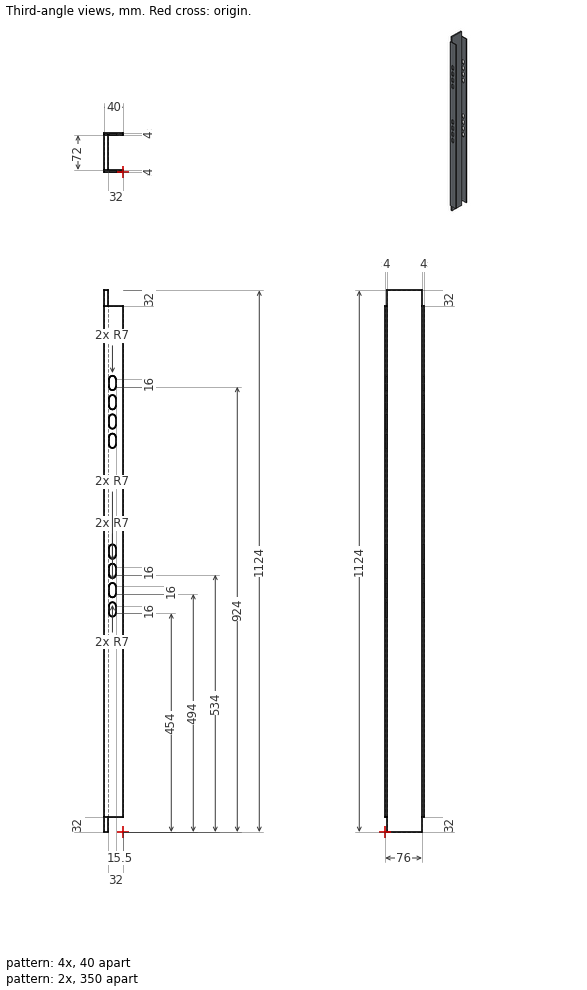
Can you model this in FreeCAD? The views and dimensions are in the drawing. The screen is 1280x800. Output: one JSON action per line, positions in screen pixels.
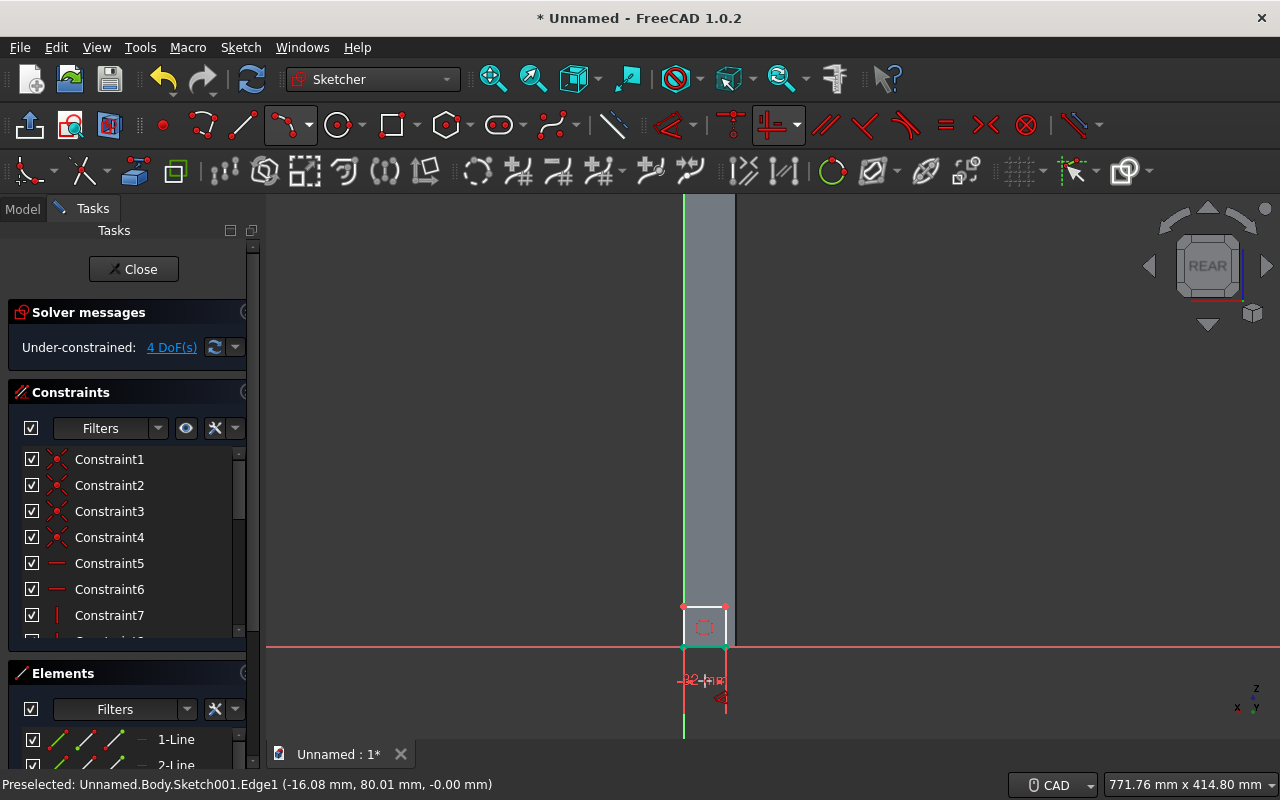
{"action": "left_click", "coordinate": [726, 635]}
{"action": "left_click", "coordinate": [760, 627]}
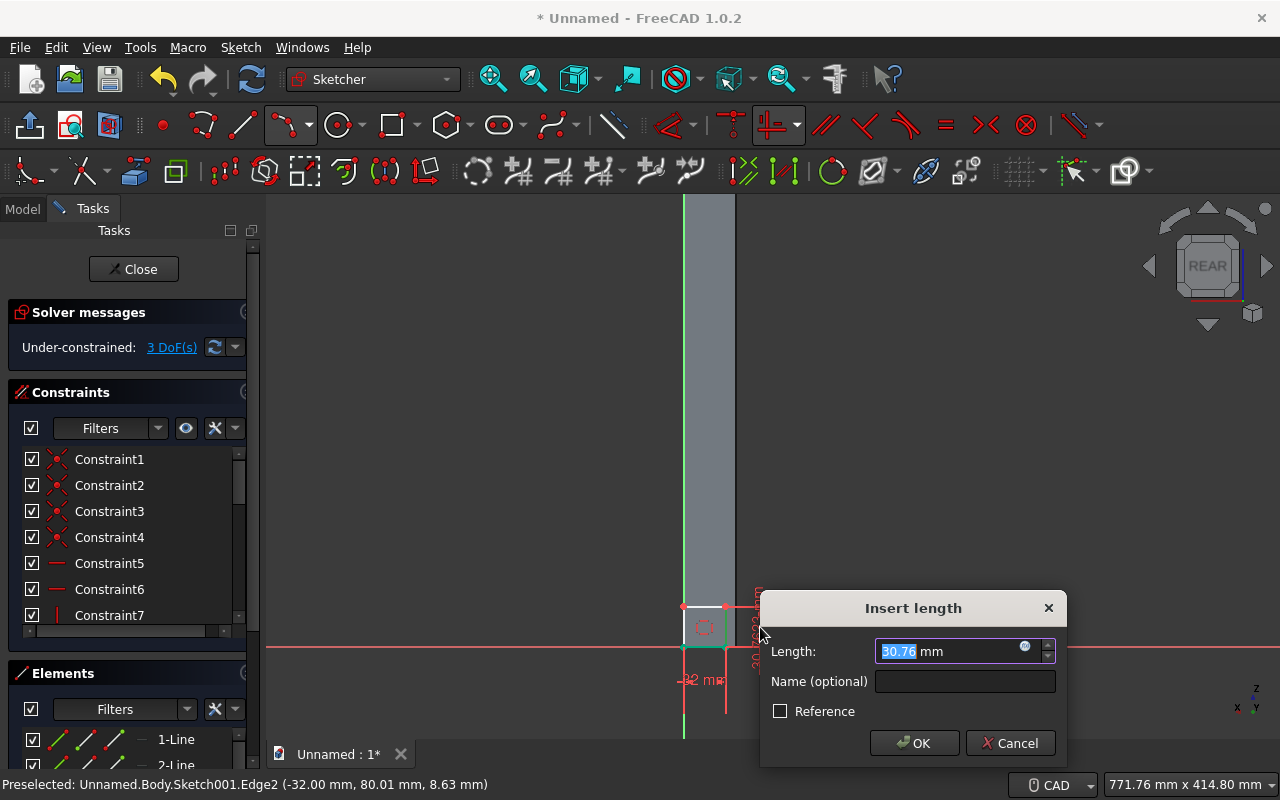
{"action": "type", "text": "32"}
{"action": "key", "text": "Return"}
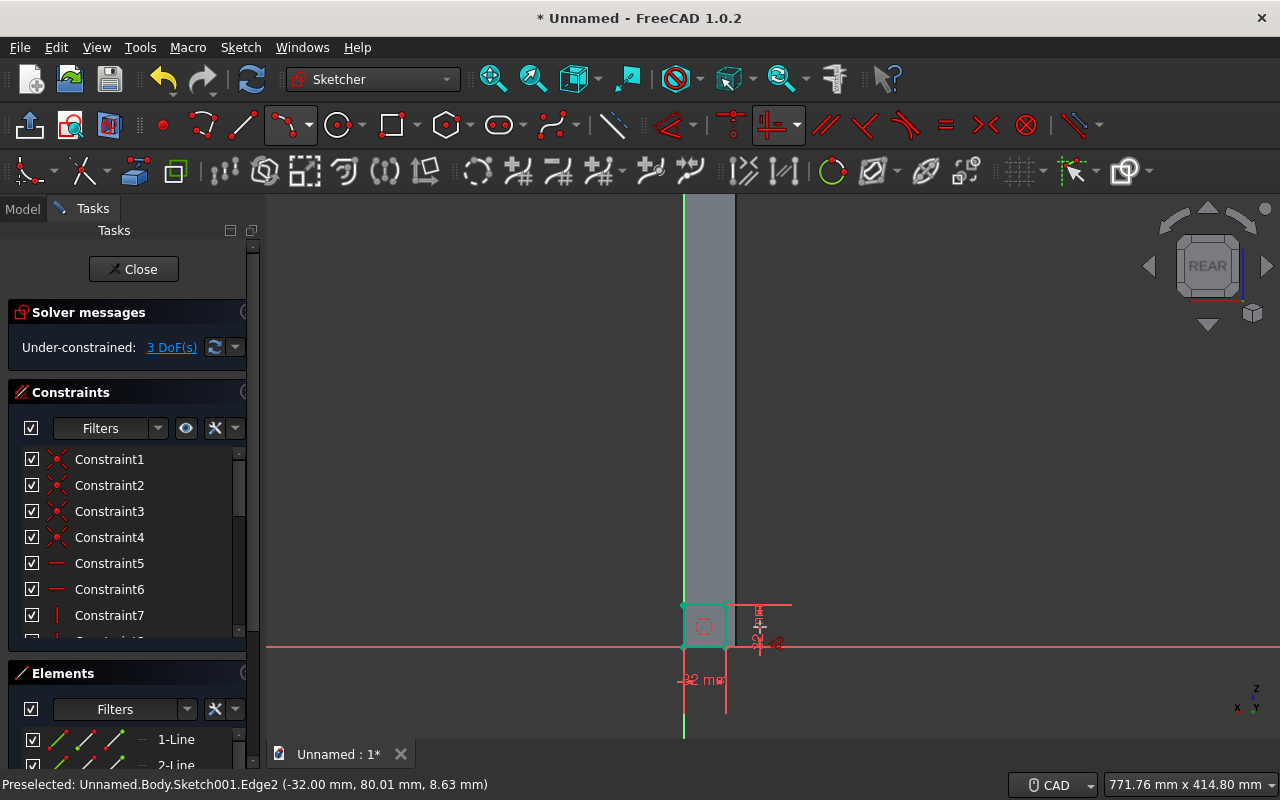
{"action": "scroll", "coordinate": [704, 649], "scroll_direction": "down", "scroll_amount": 7}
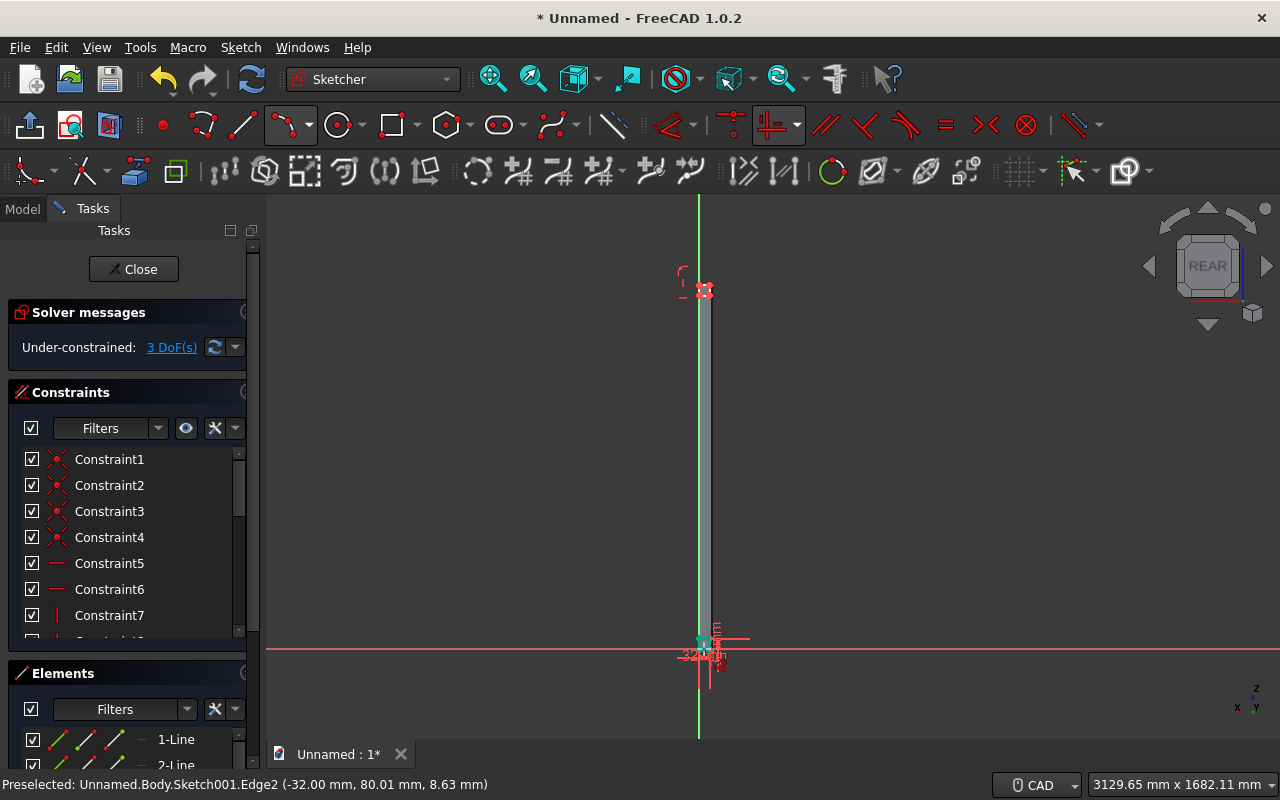
{"action": "scroll", "coordinate": [699, 289], "scroll_direction": "up", "scroll_amount": 8}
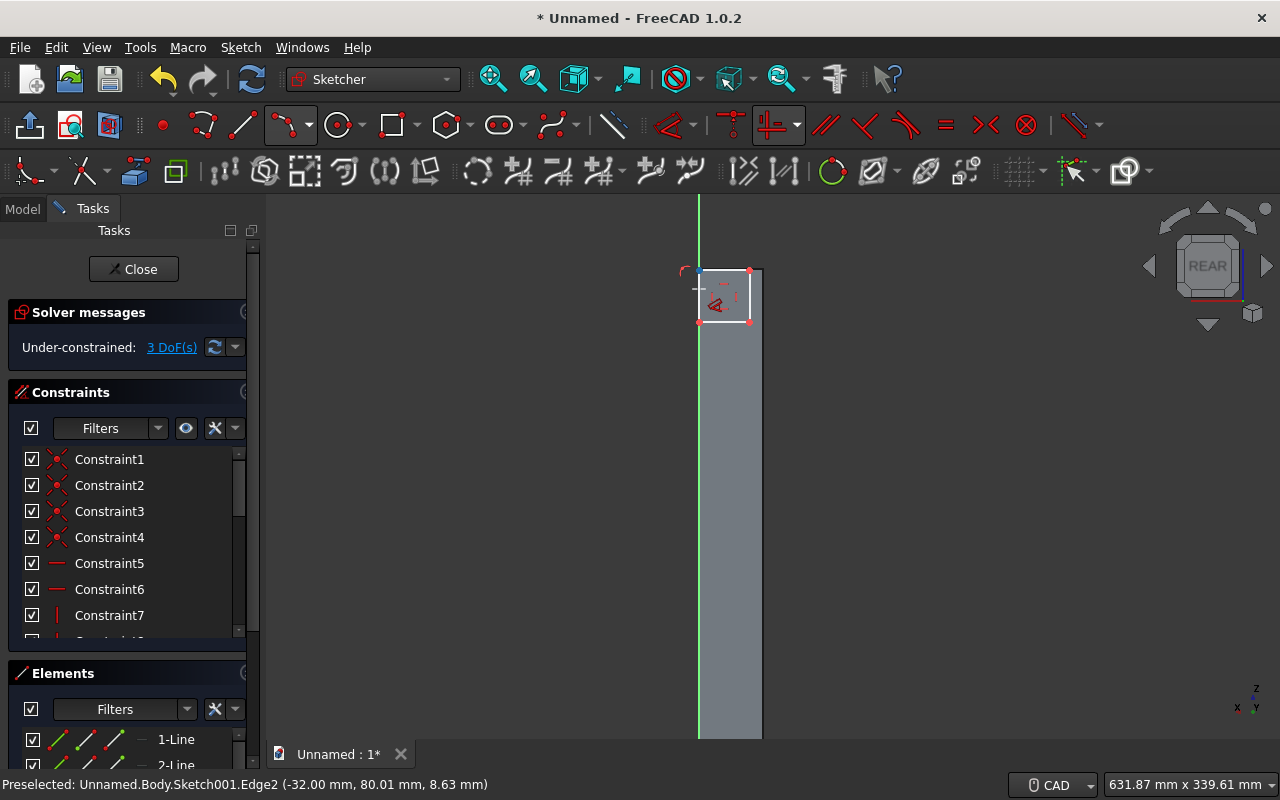
{"action": "left_click", "coordinate": [699, 286]}
{"action": "left_click", "coordinate": [665, 296]}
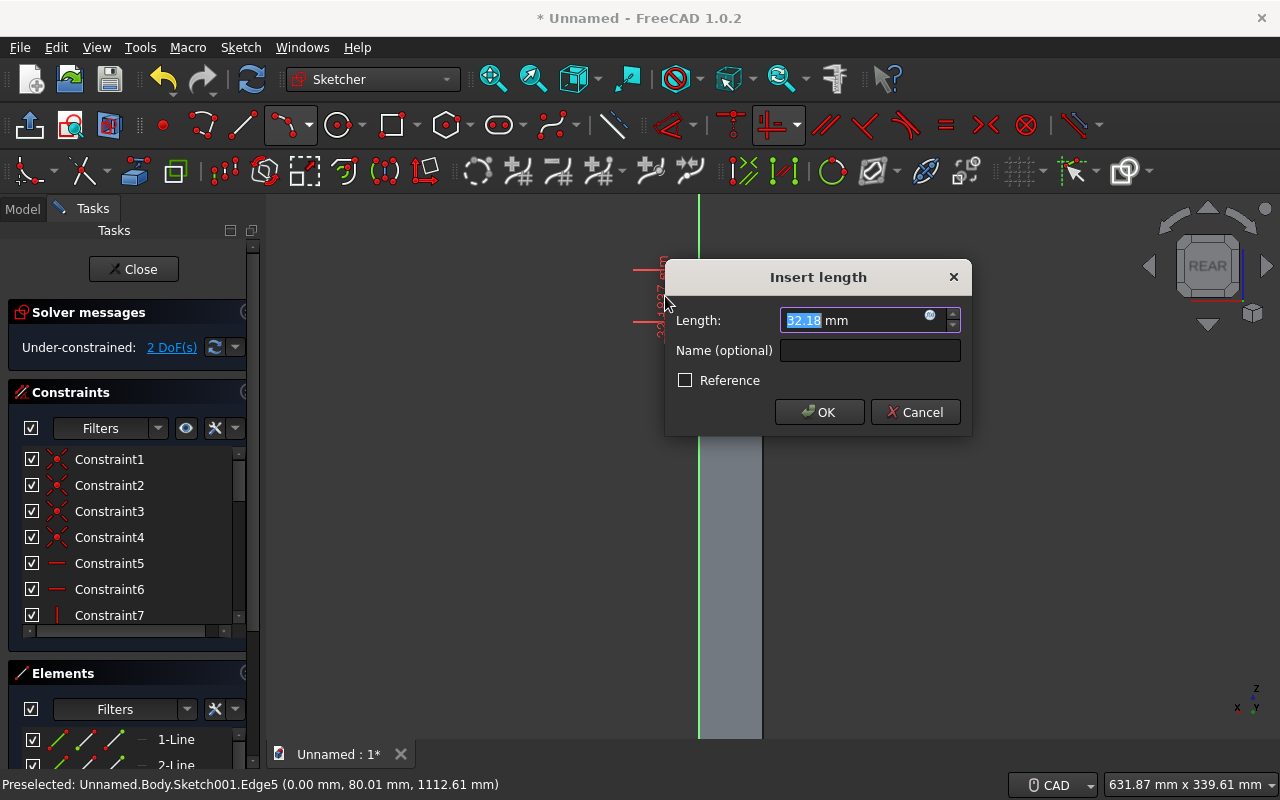
{"action": "type", "text": "32"}
{"action": "key", "text": "Return"}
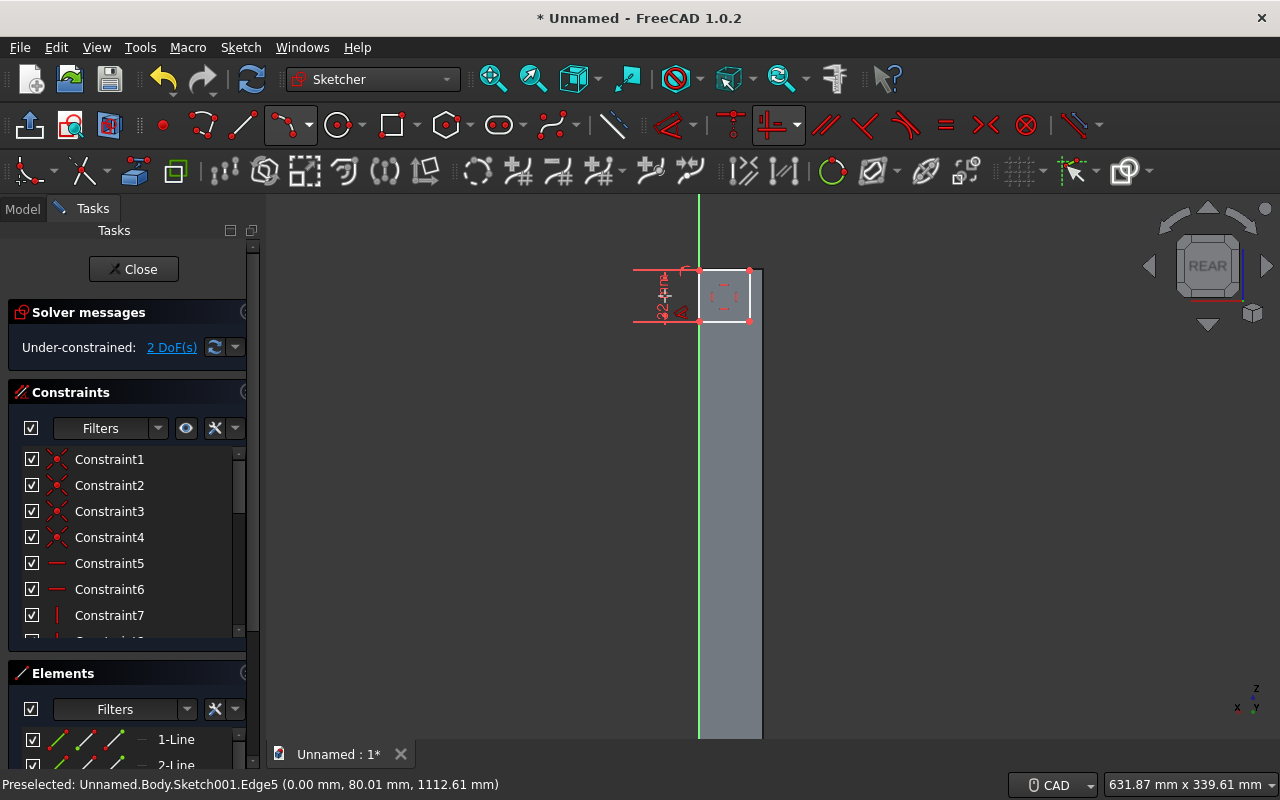
{"action": "left_click", "coordinate": [714, 322]}
{"action": "left_click", "coordinate": [736, 288]}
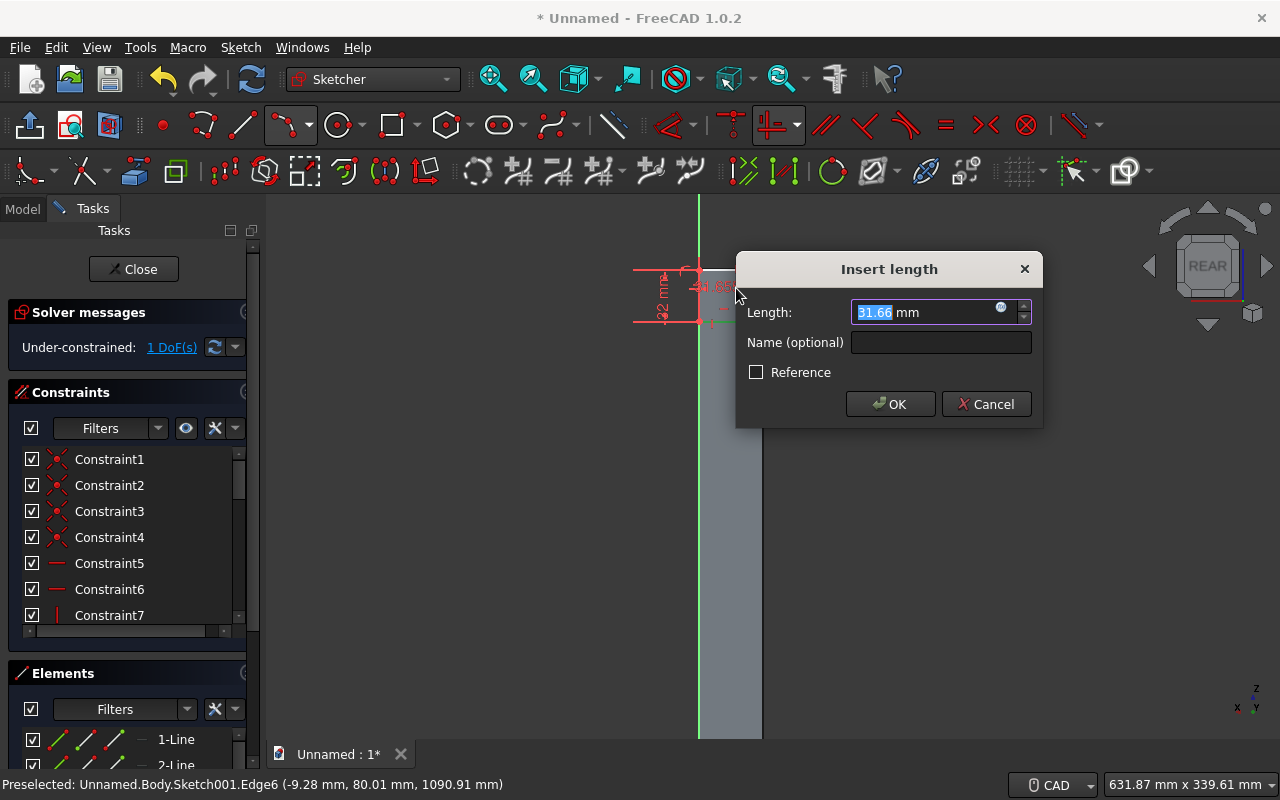
{"action": "type", "text": "32"}
{"action": "key", "text": "Return"}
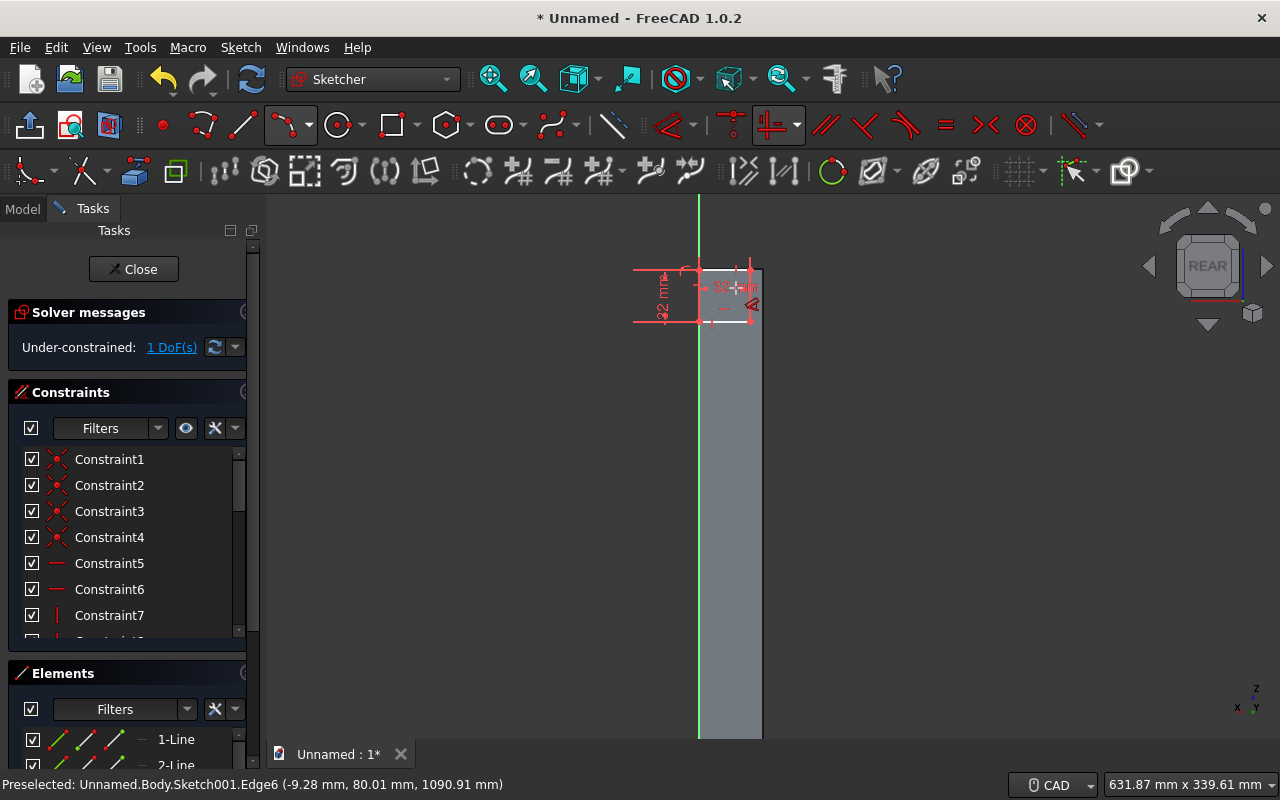
{"action": "scroll", "coordinate": [699, 288], "scroll_direction": "down", "scroll_amount": 8}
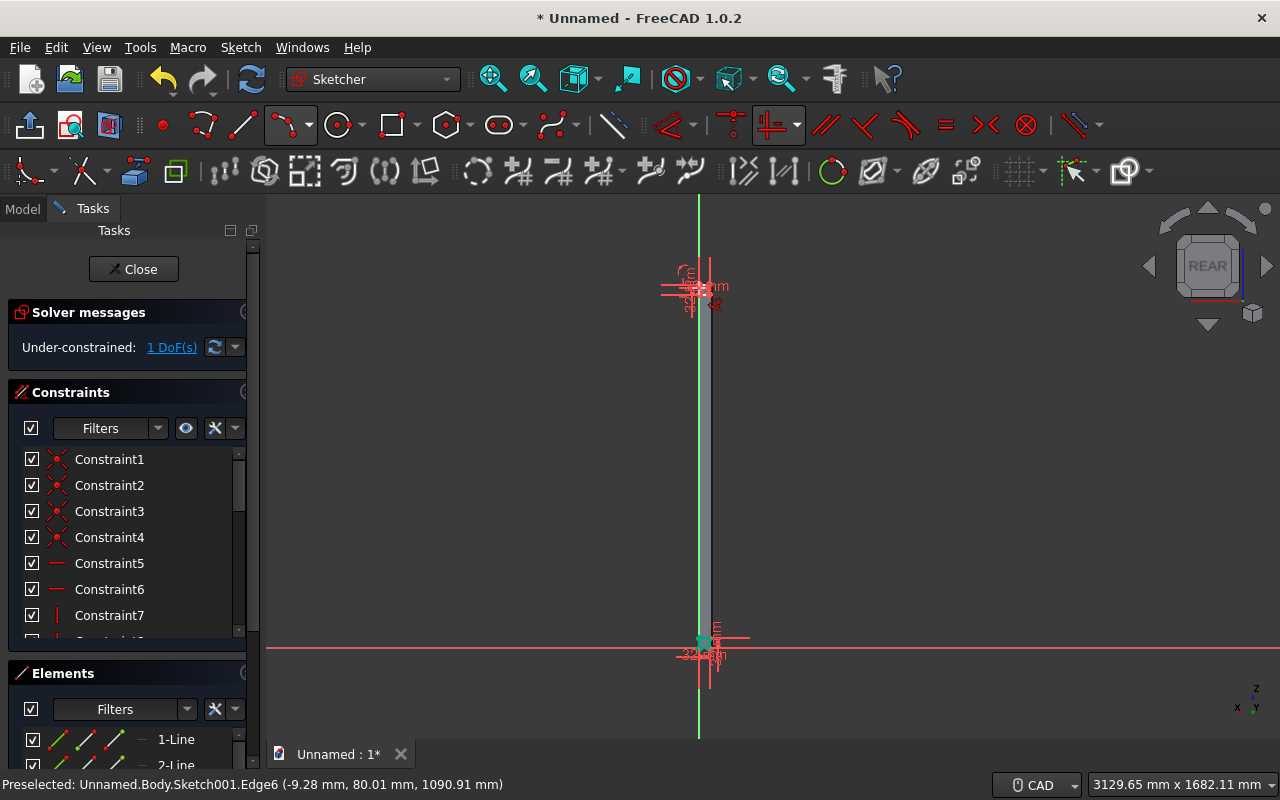
{"action": "left_click", "coordinate": [699, 285]}
{"action": "left_click", "coordinate": [665, 467]}